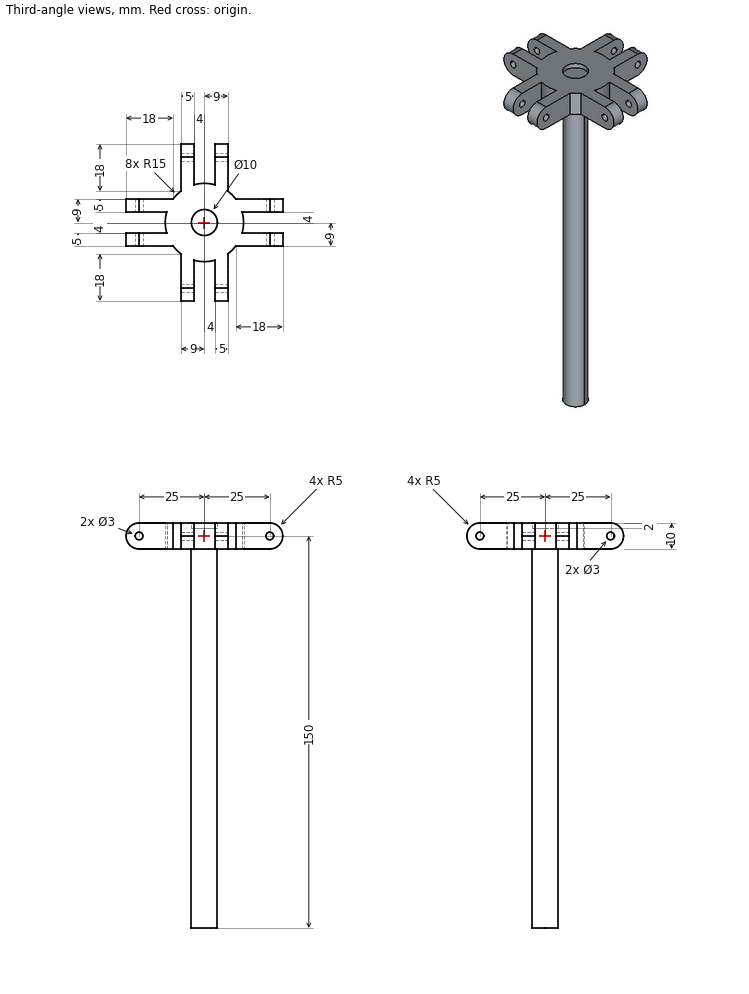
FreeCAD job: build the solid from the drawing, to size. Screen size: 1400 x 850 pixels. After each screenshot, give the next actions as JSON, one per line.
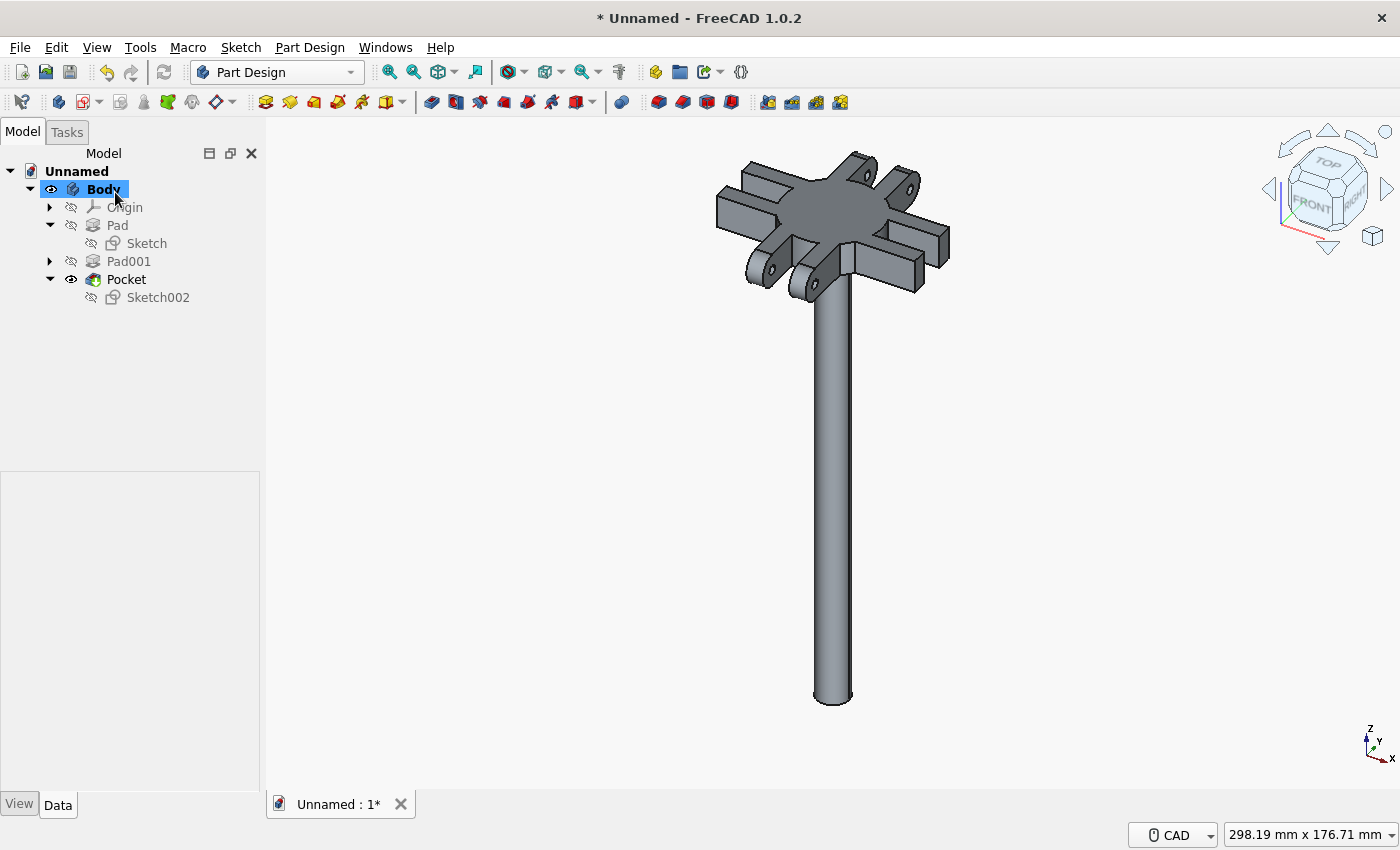
{"action": "key", "text": "4"}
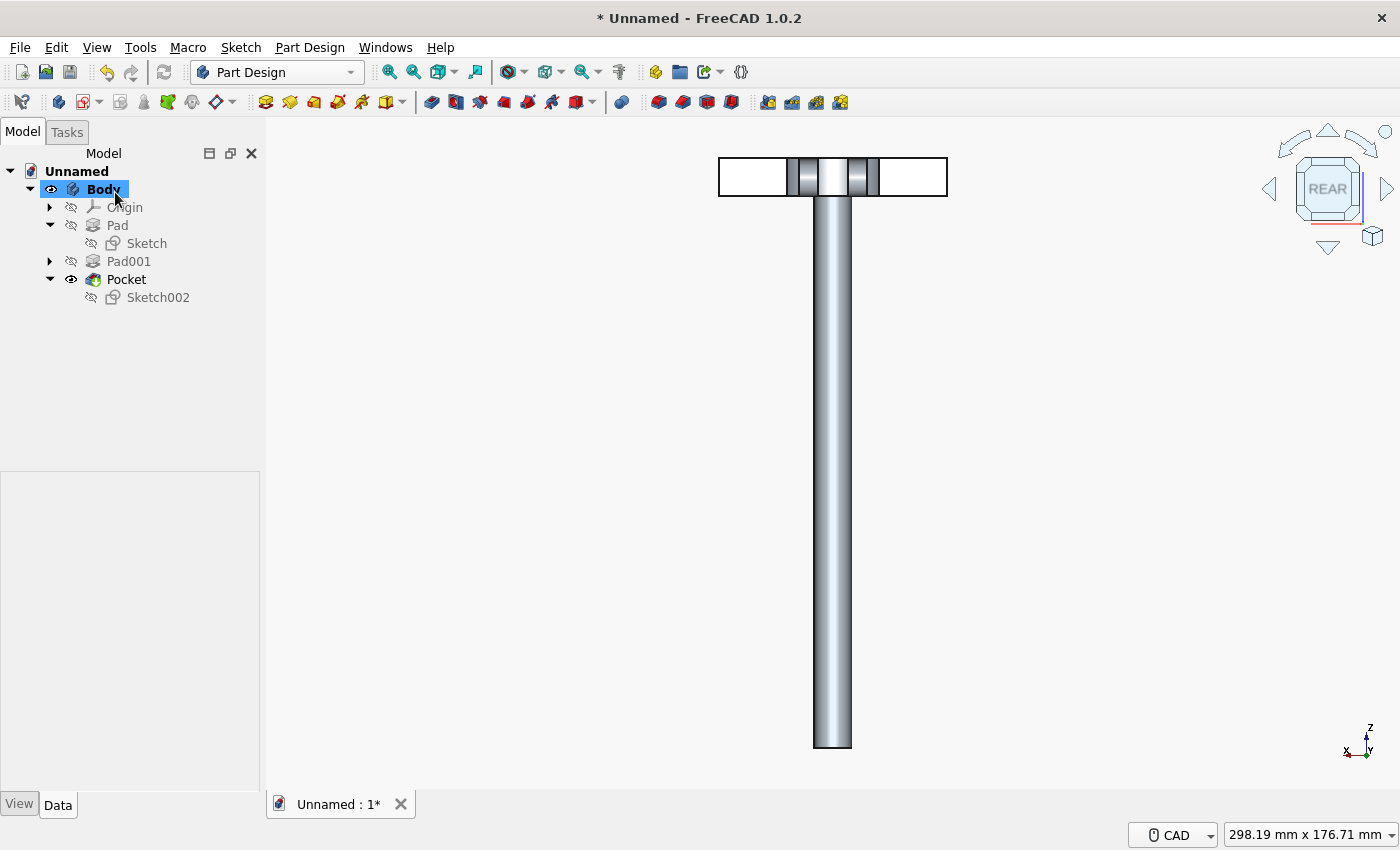
{"action": "left_click", "coordinate": [743, 176]}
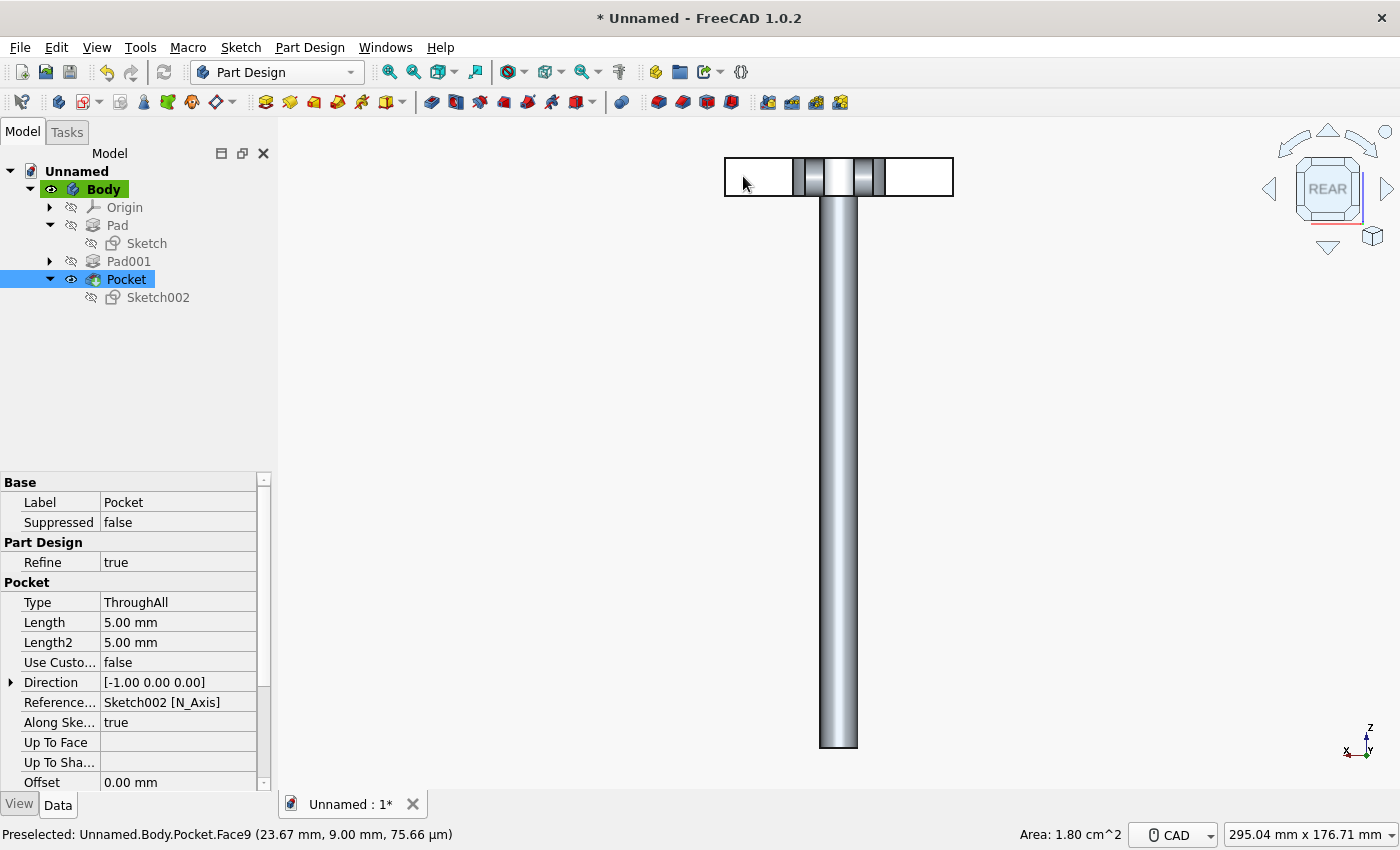
{"action": "left_click", "coordinate": [84, 102]}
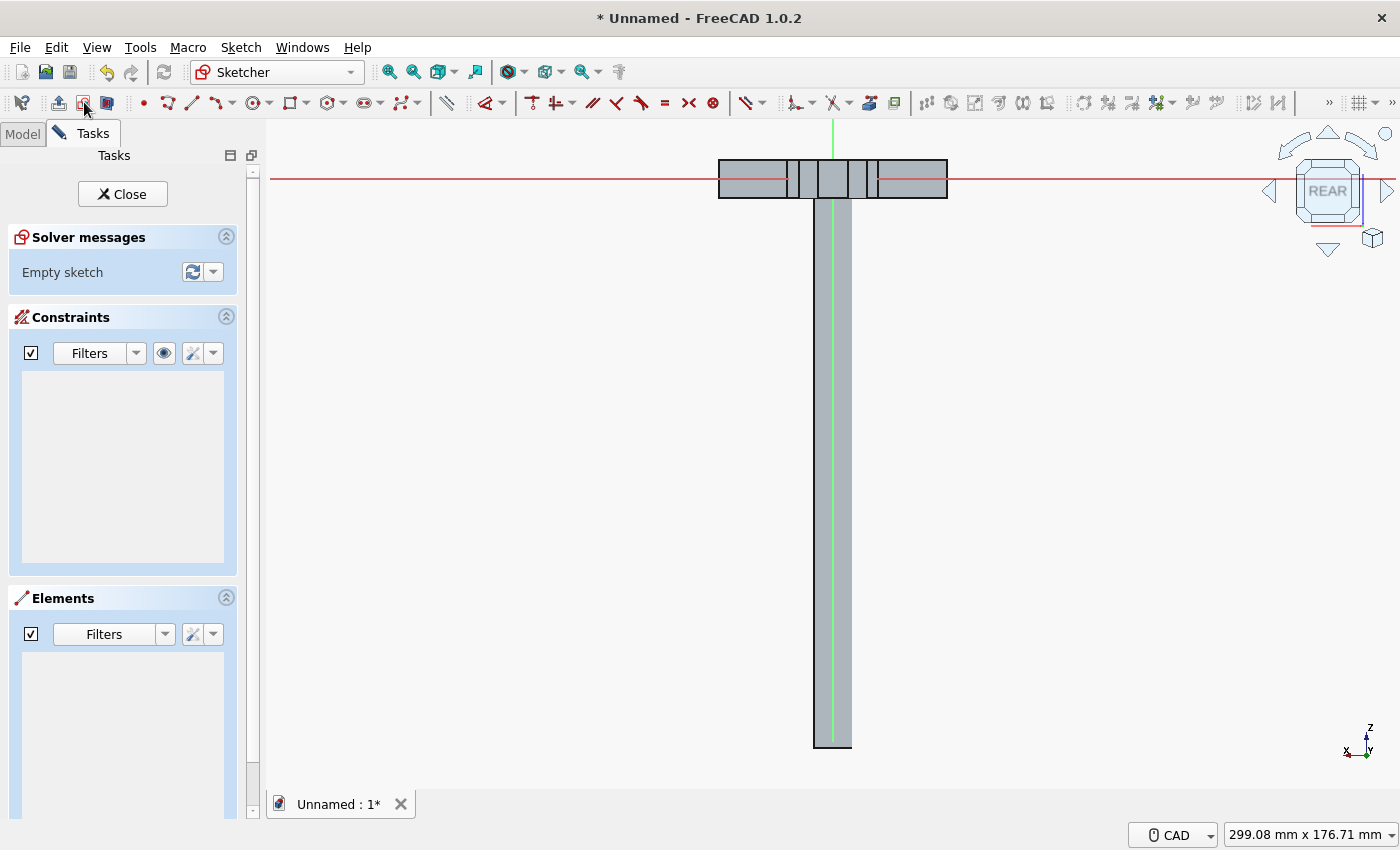
{"action": "left_click", "coordinate": [108, 104]}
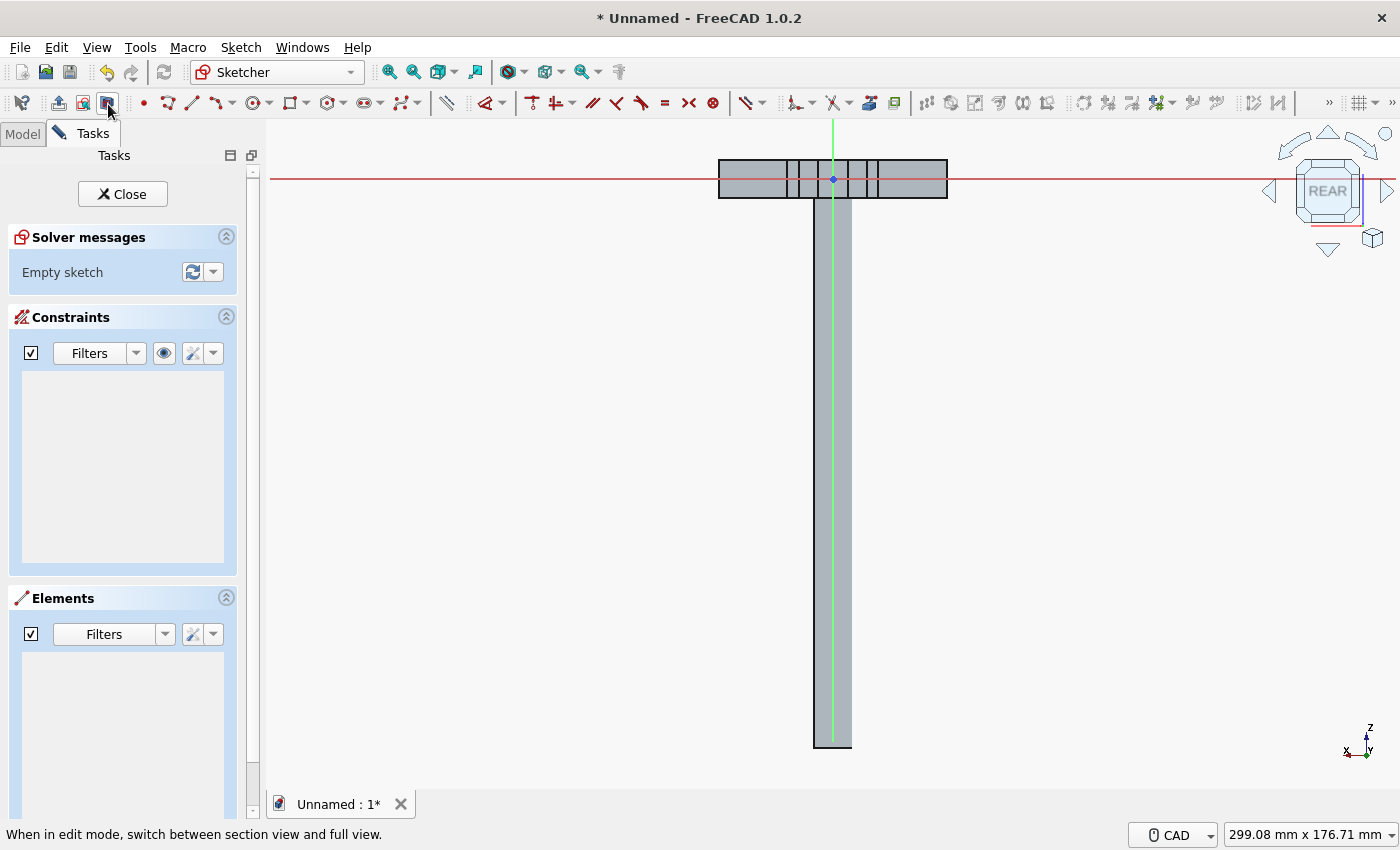
{"action": "scroll", "coordinate": [873, 147], "scroll_direction": "up", "scroll_amount": 5}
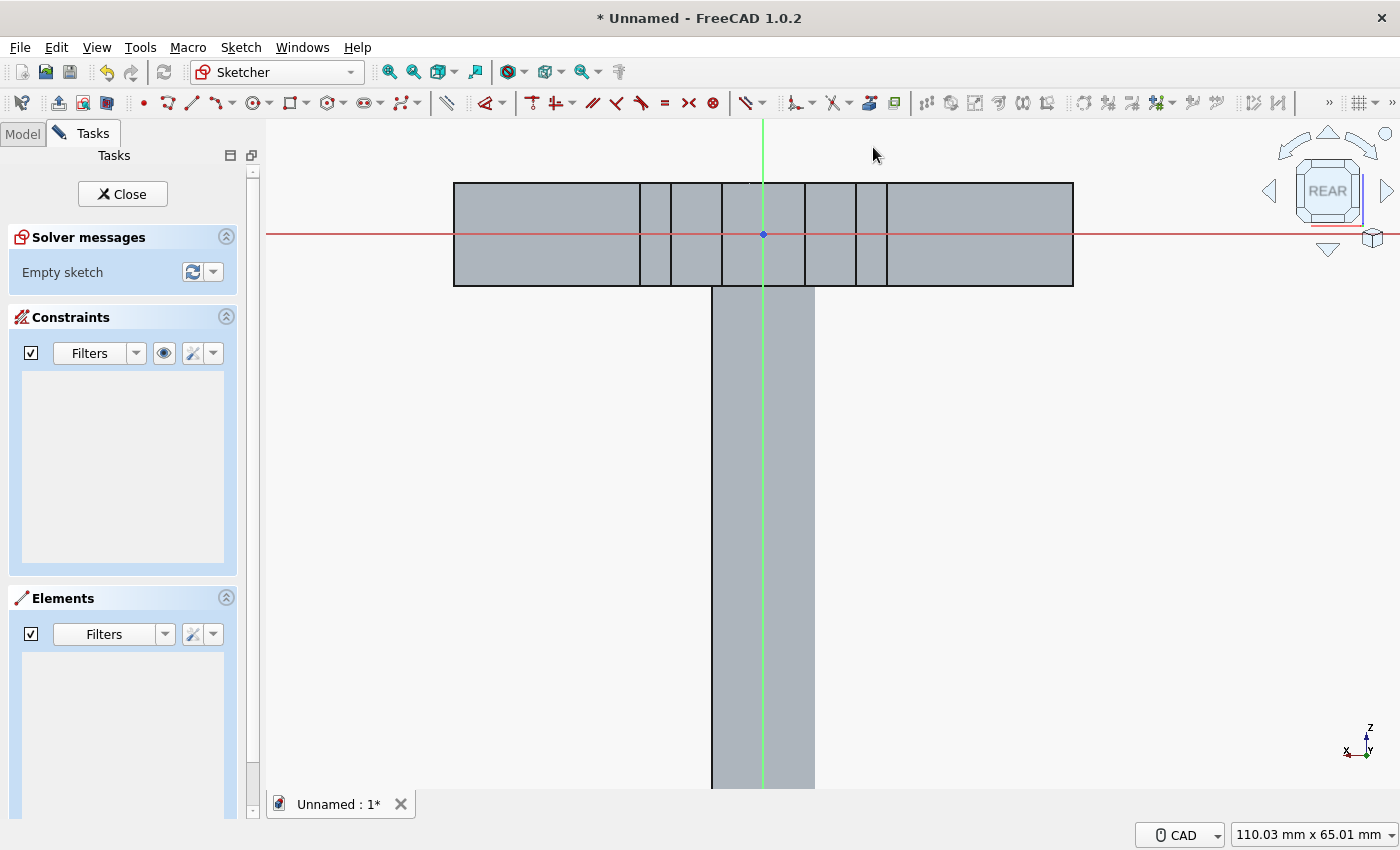
{"action": "key", "text": "g m"}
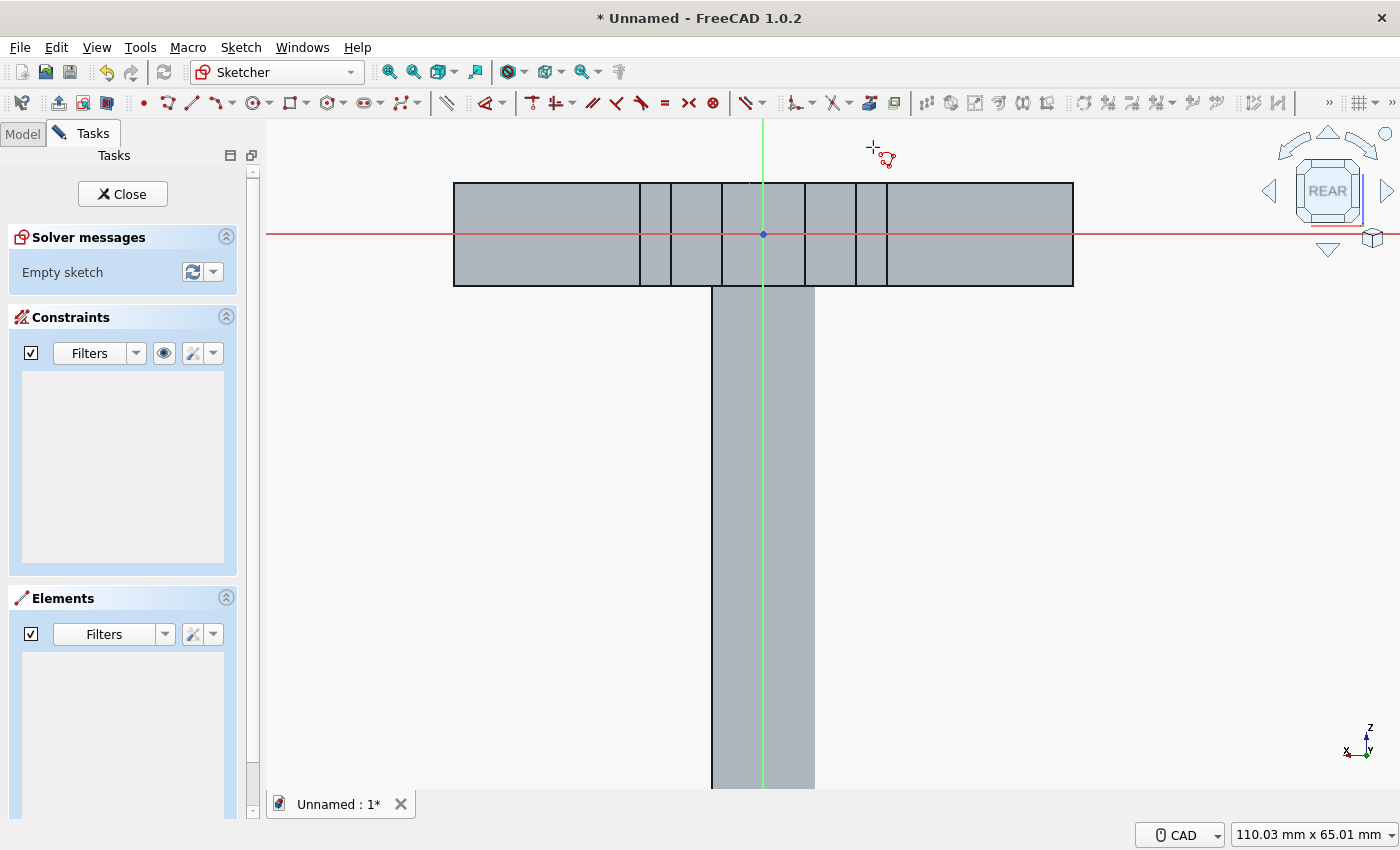
{"action": "left_click", "coordinate": [506, 183]}
{"action": "left_click", "coordinate": [454, 183]}
{"action": "left_click", "coordinate": [454, 234]}
{"action": "right_click", "coordinate": [454, 234]}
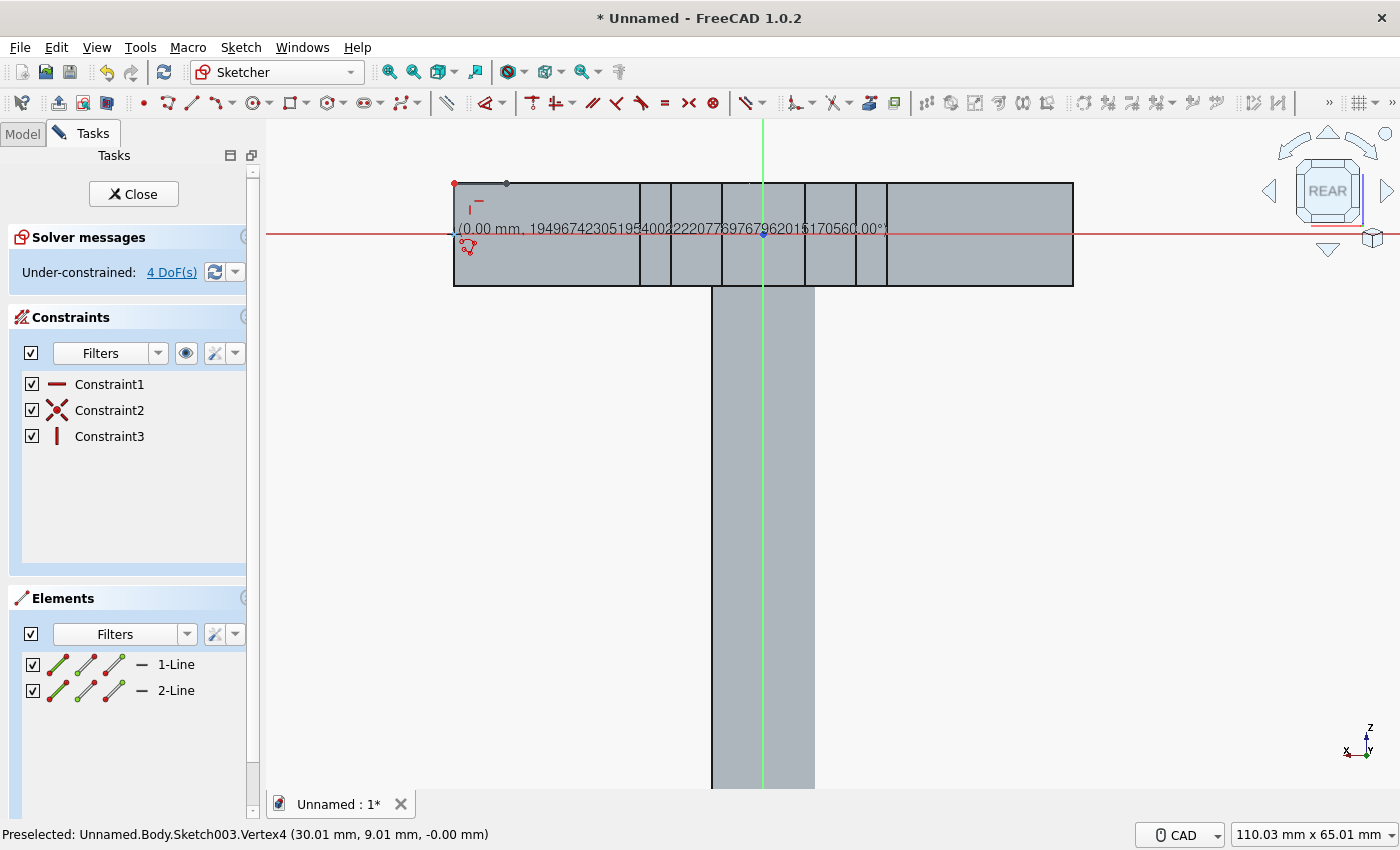
{"action": "key", "text": "g 3 a"}